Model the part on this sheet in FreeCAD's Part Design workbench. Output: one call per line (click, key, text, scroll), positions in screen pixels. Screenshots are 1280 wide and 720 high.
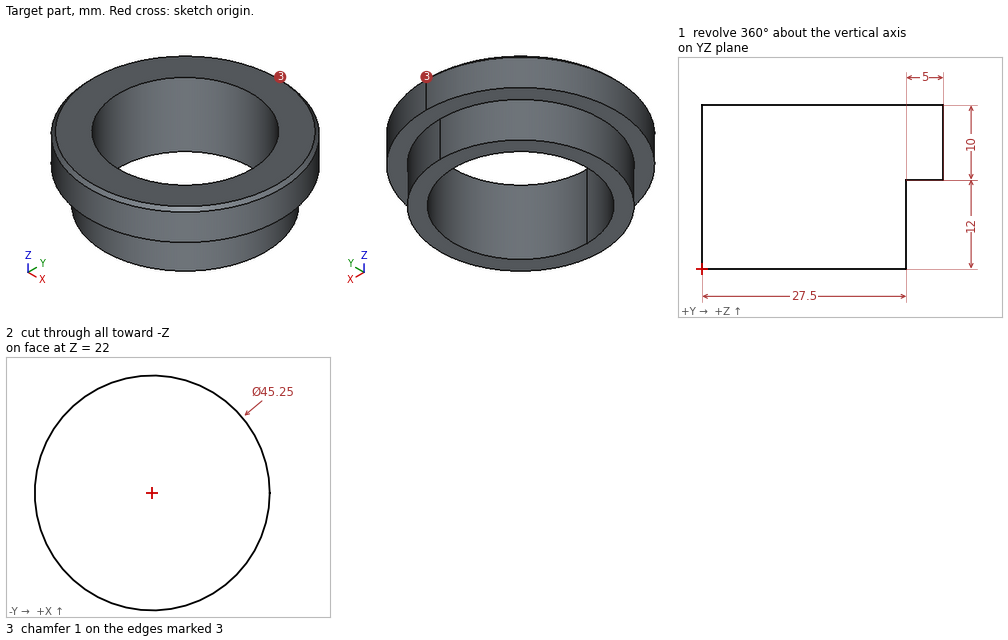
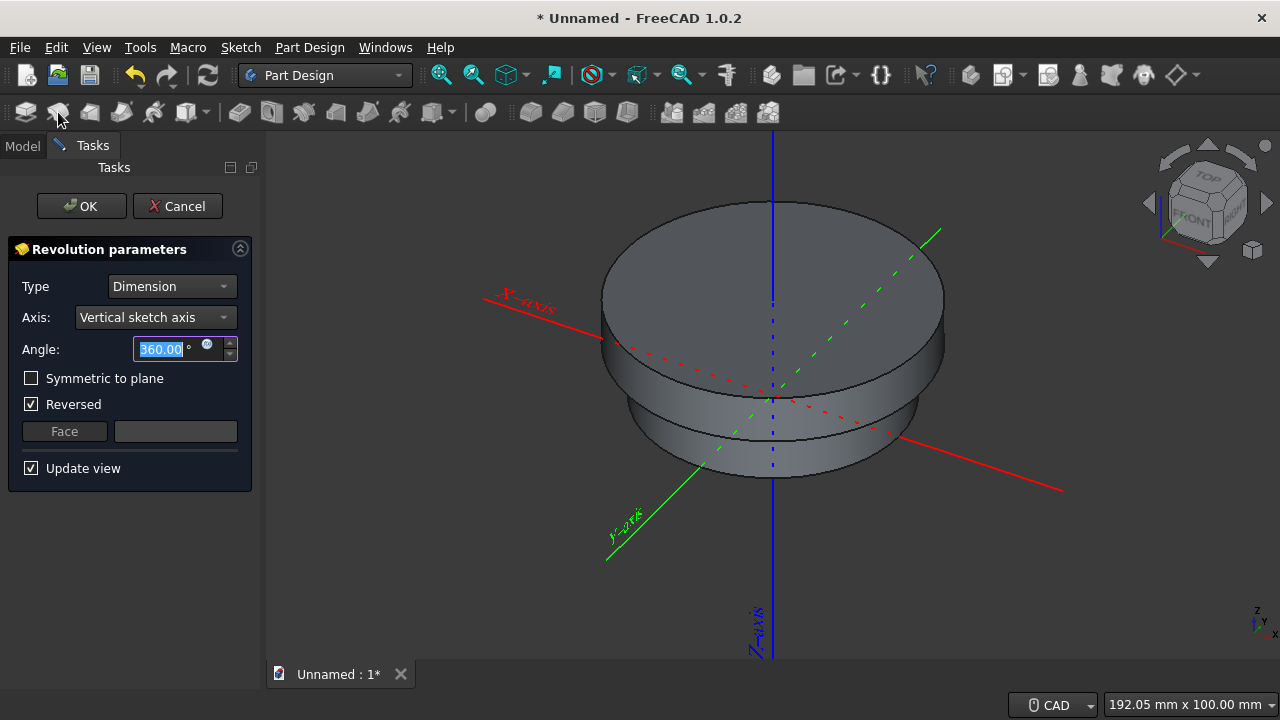
click(82, 206)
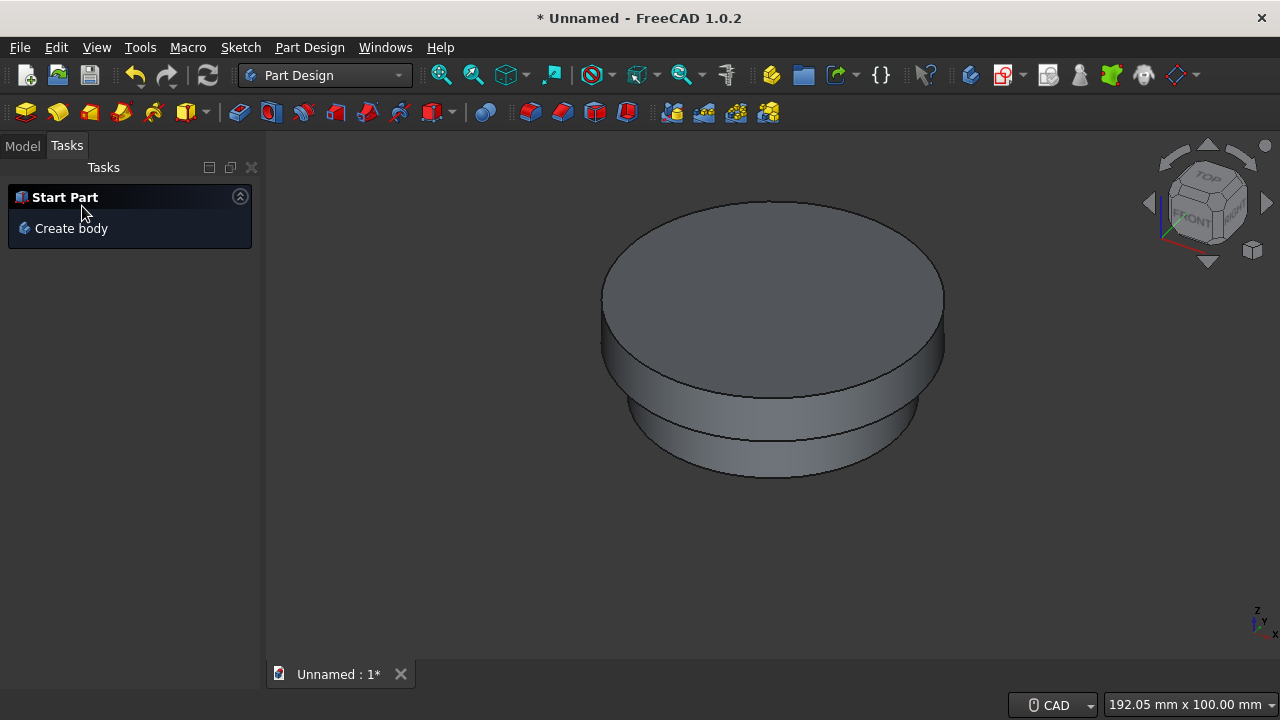
click(773, 299)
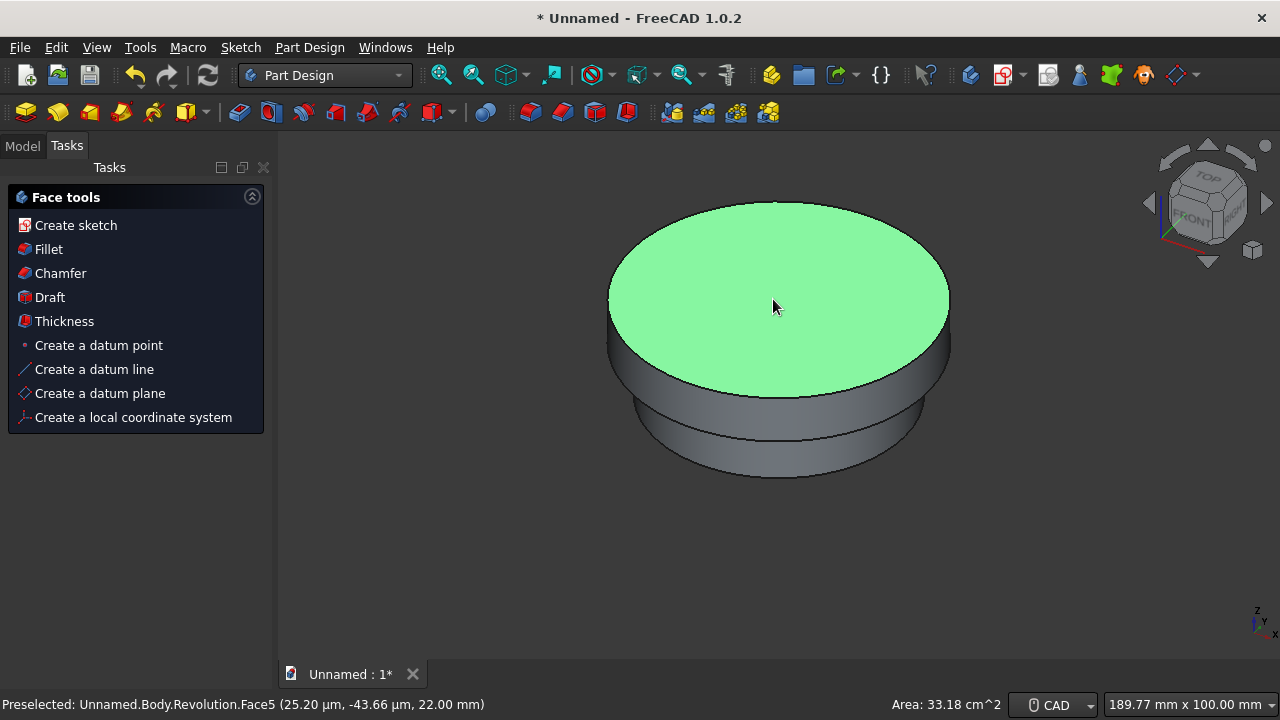
click(1004, 76)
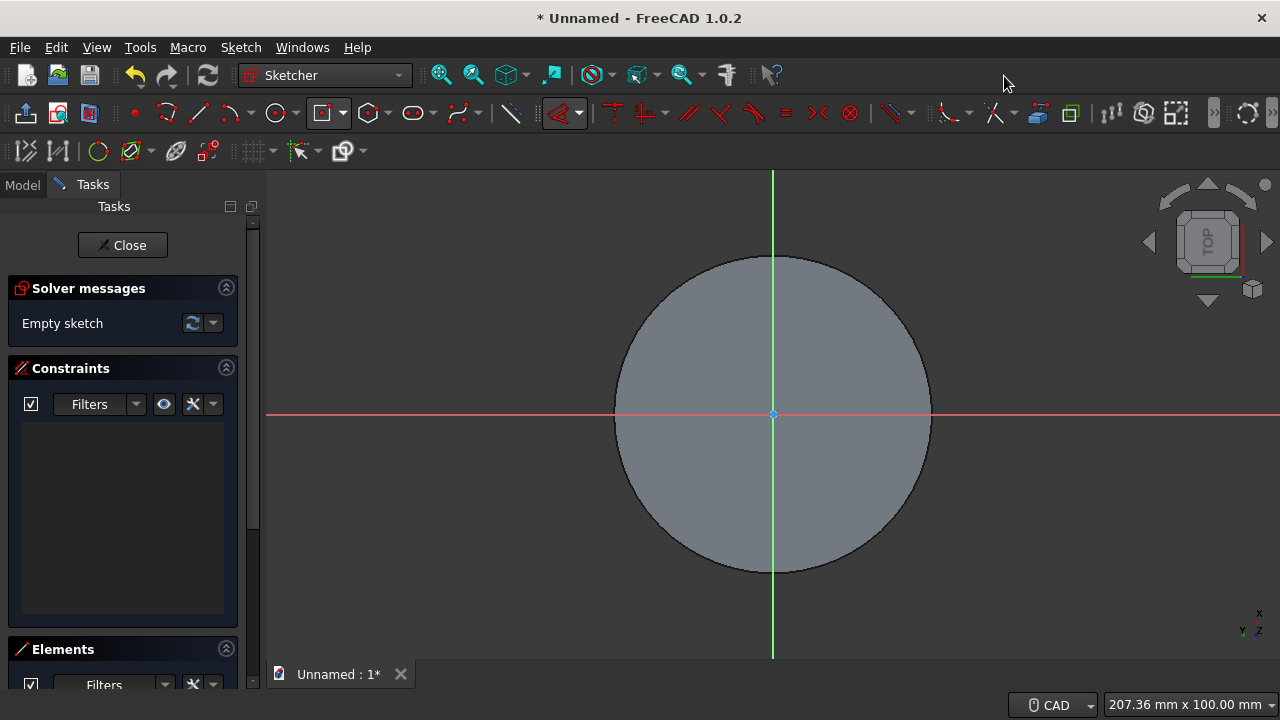
scroll(912, 414, up, 2)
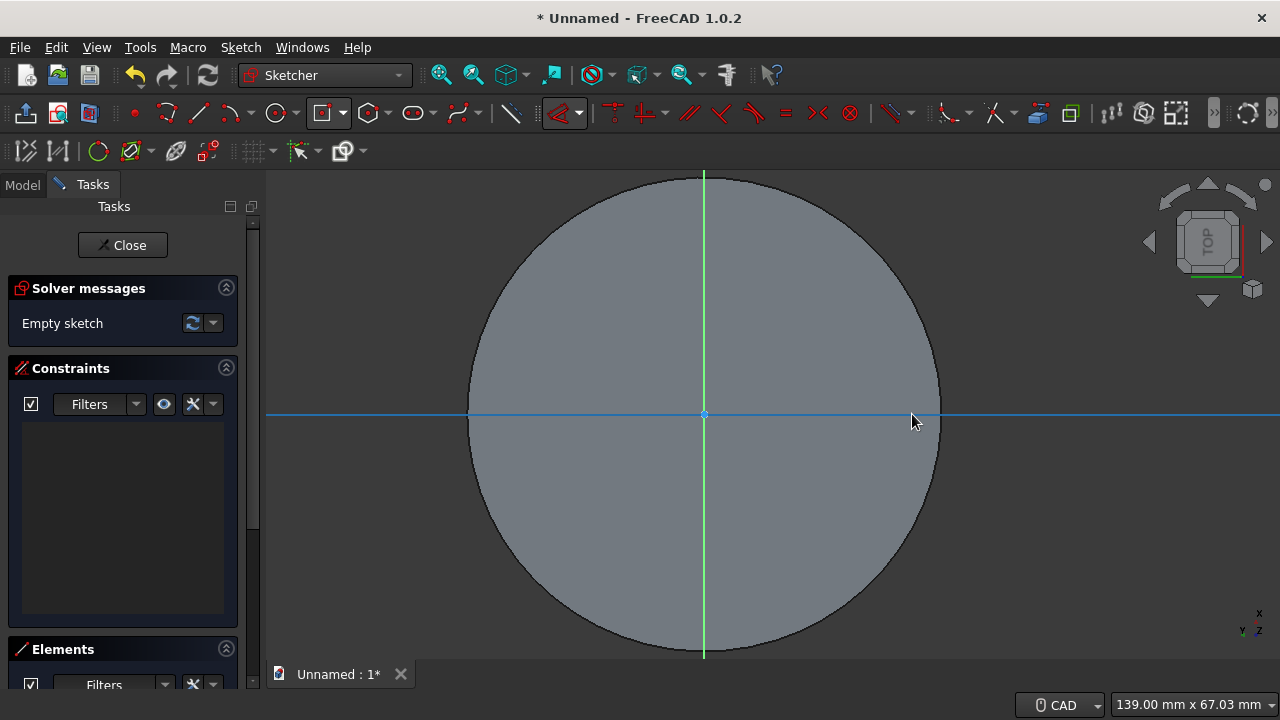
click(276, 114)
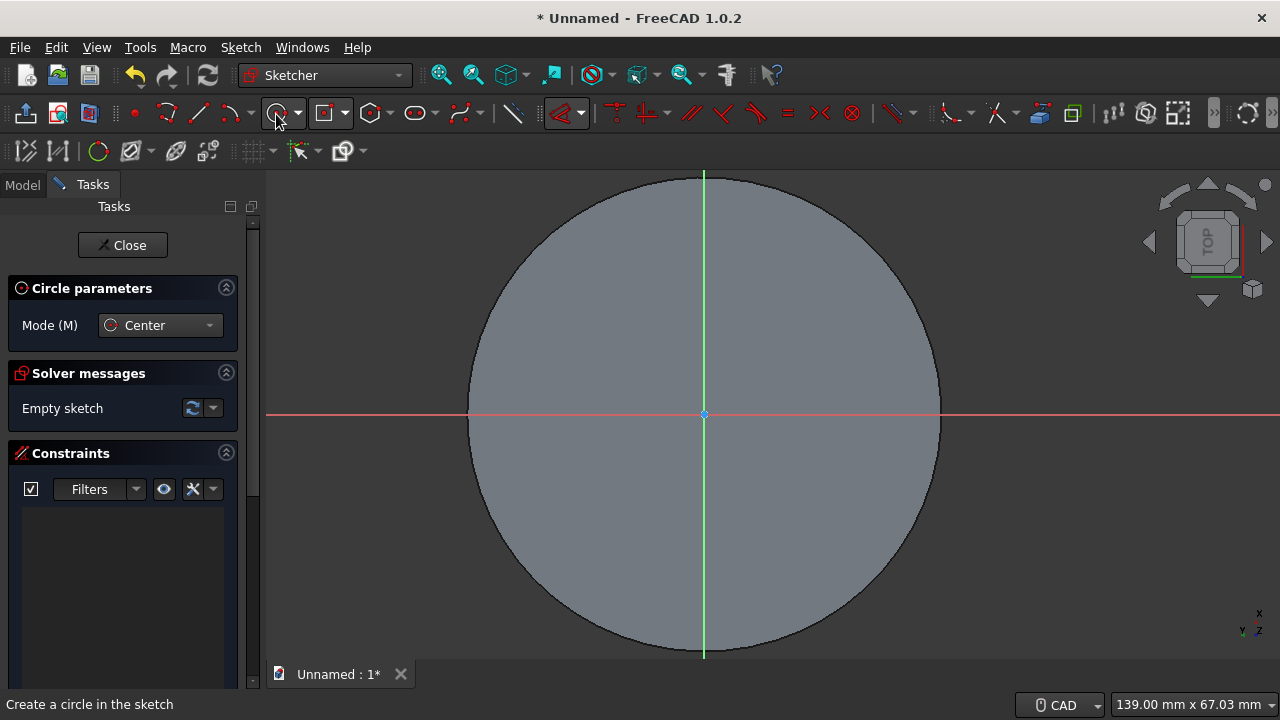
click(704, 415)
move(821, 298)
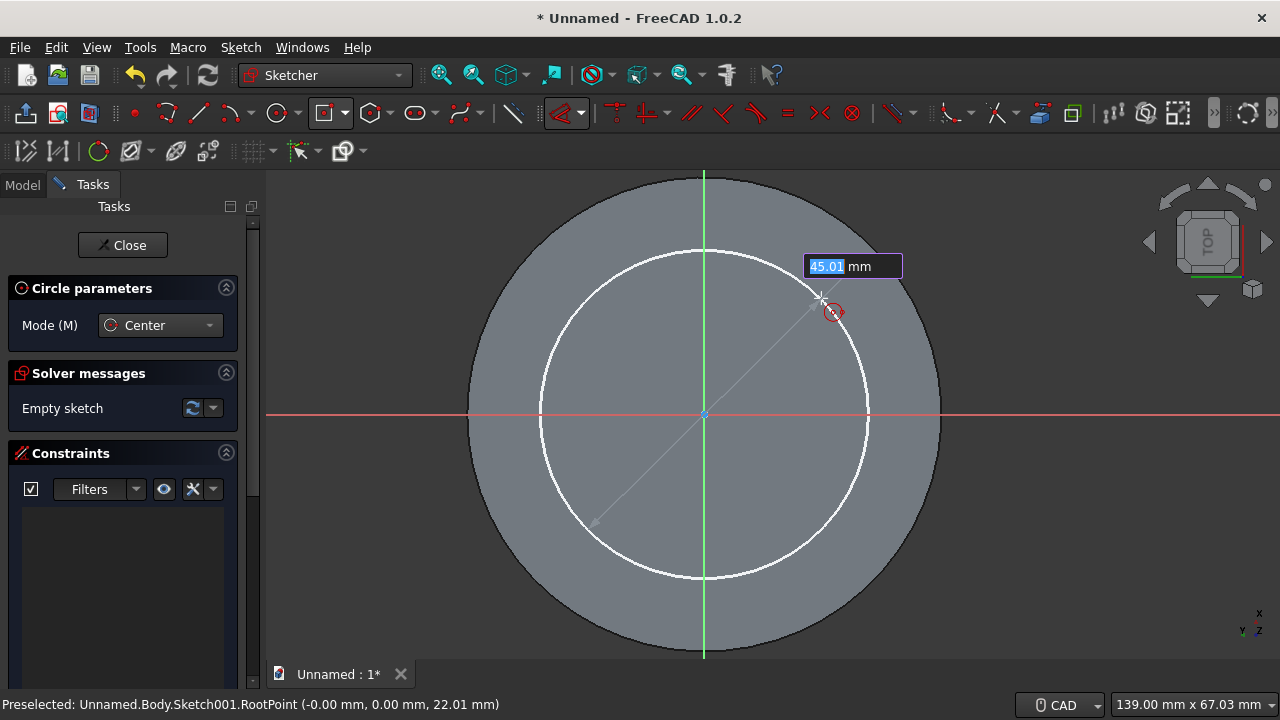
text(45.25)
key(Return)
key(Escape)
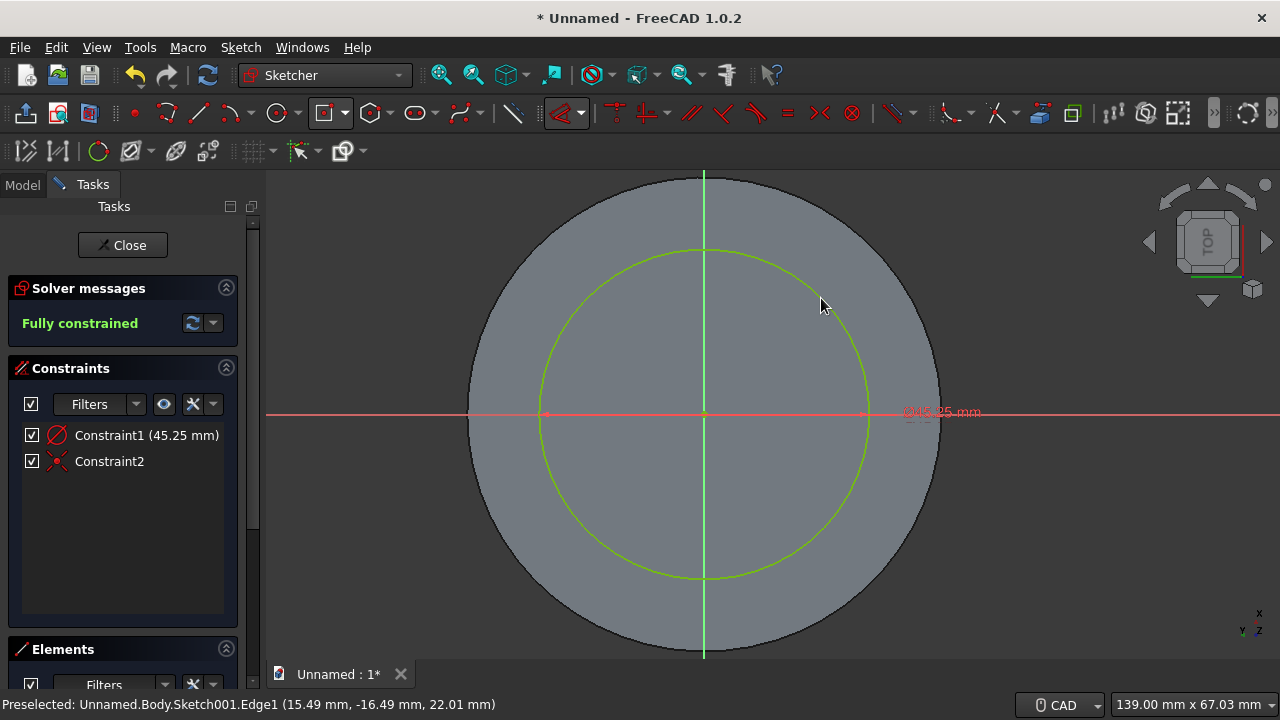
click(123, 245)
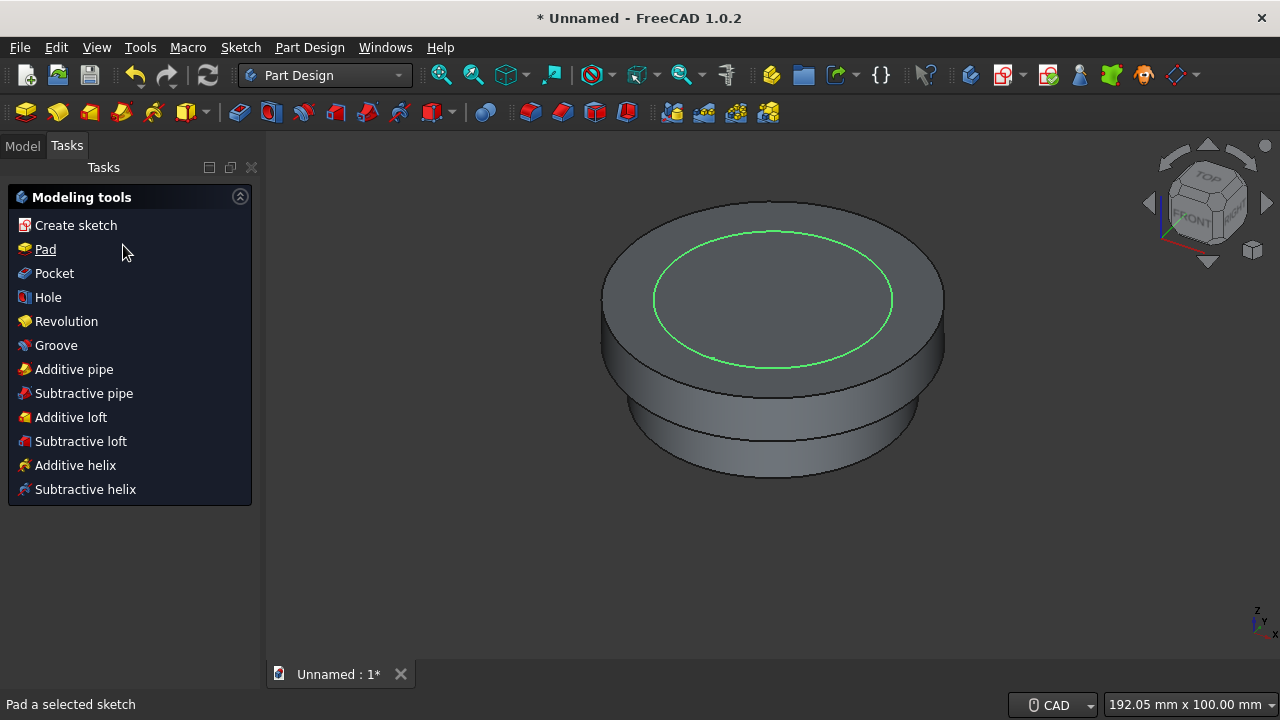
click(240, 112)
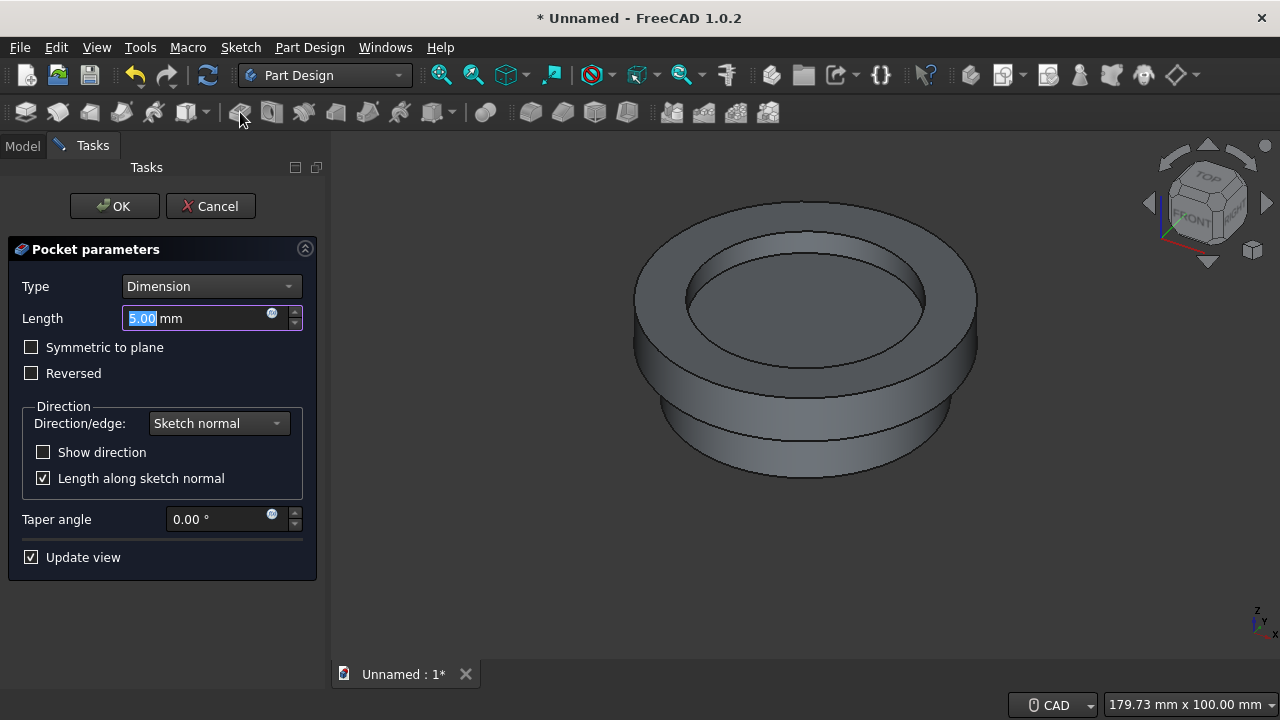
click(212, 286)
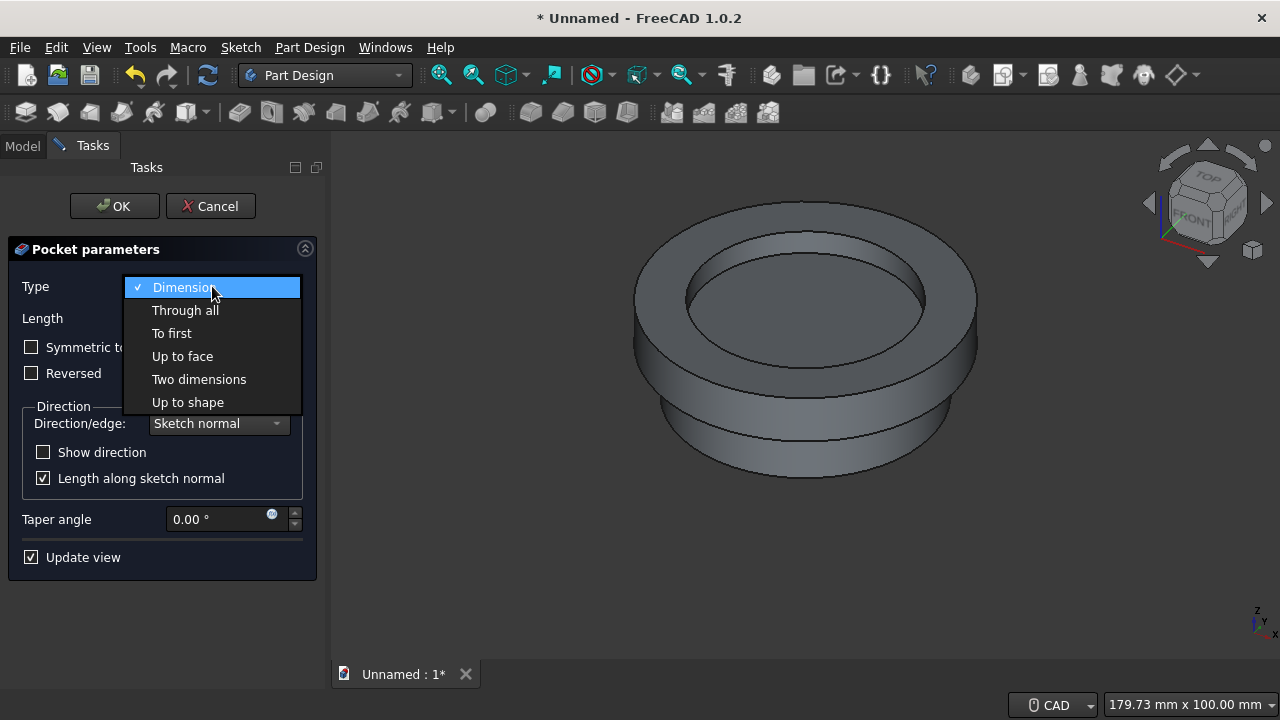
click(212, 310)